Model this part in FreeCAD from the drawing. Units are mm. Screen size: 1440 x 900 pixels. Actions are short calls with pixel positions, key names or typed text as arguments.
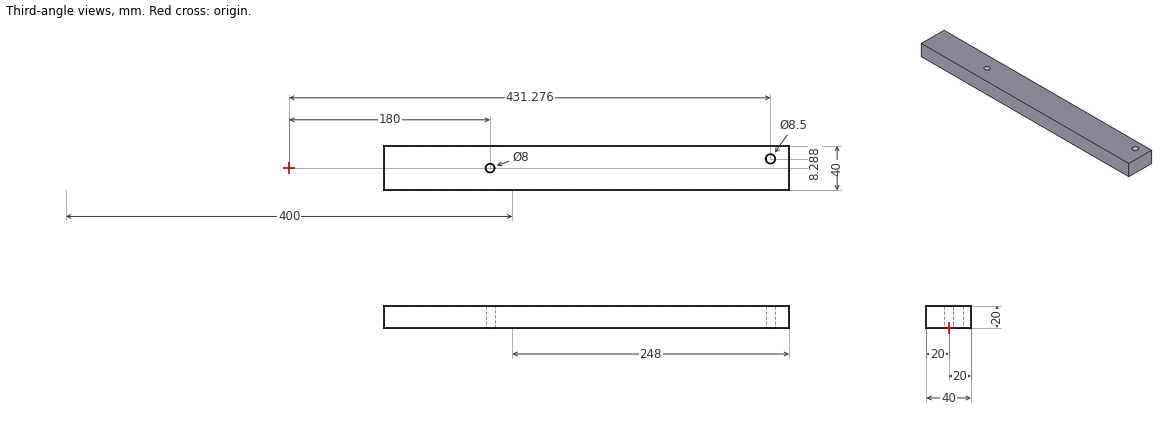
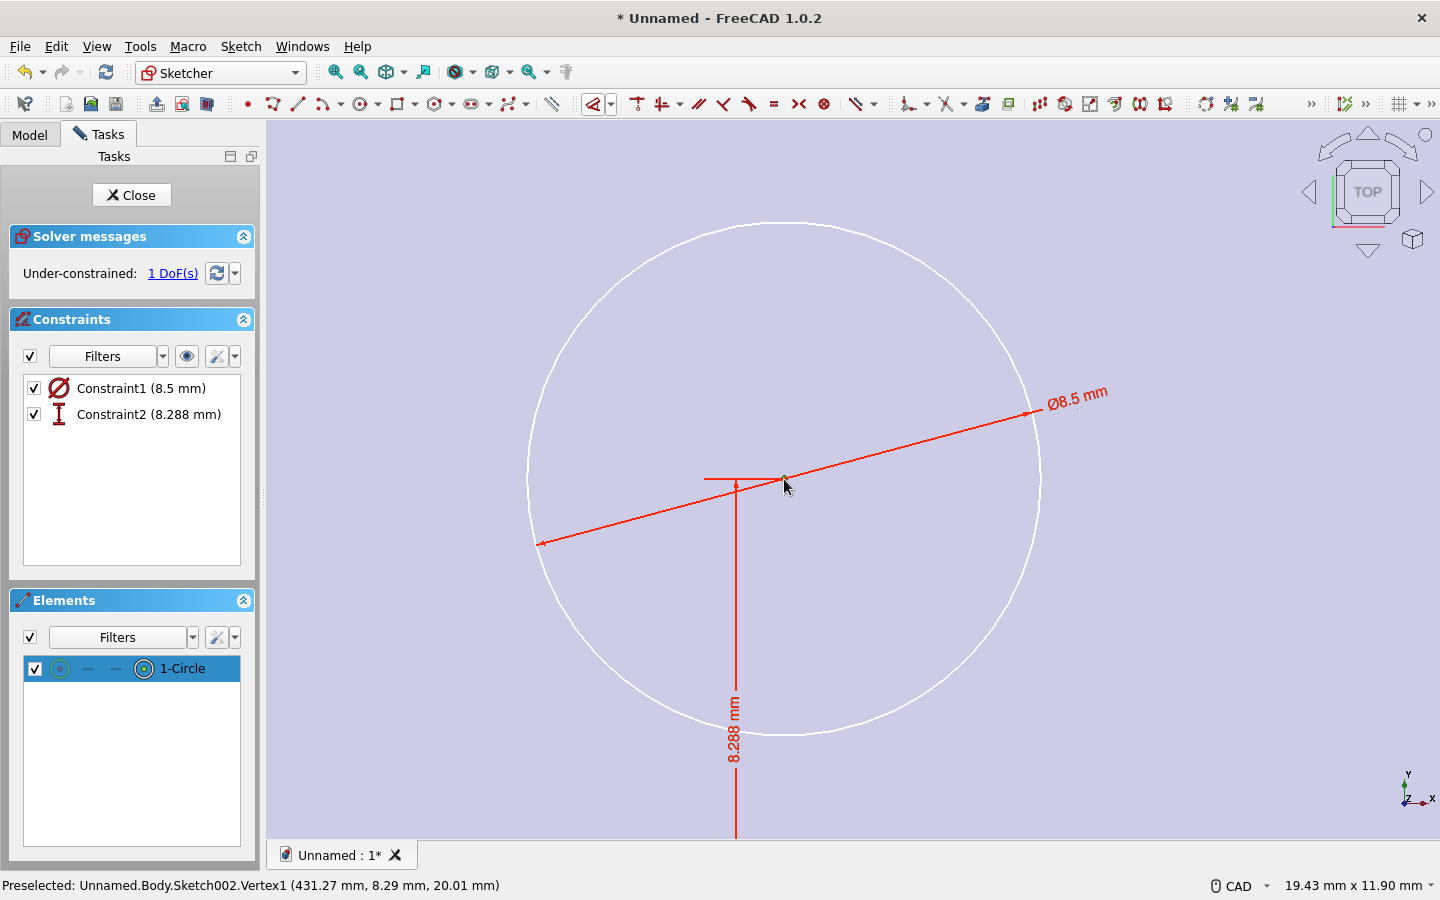
click(610, 104)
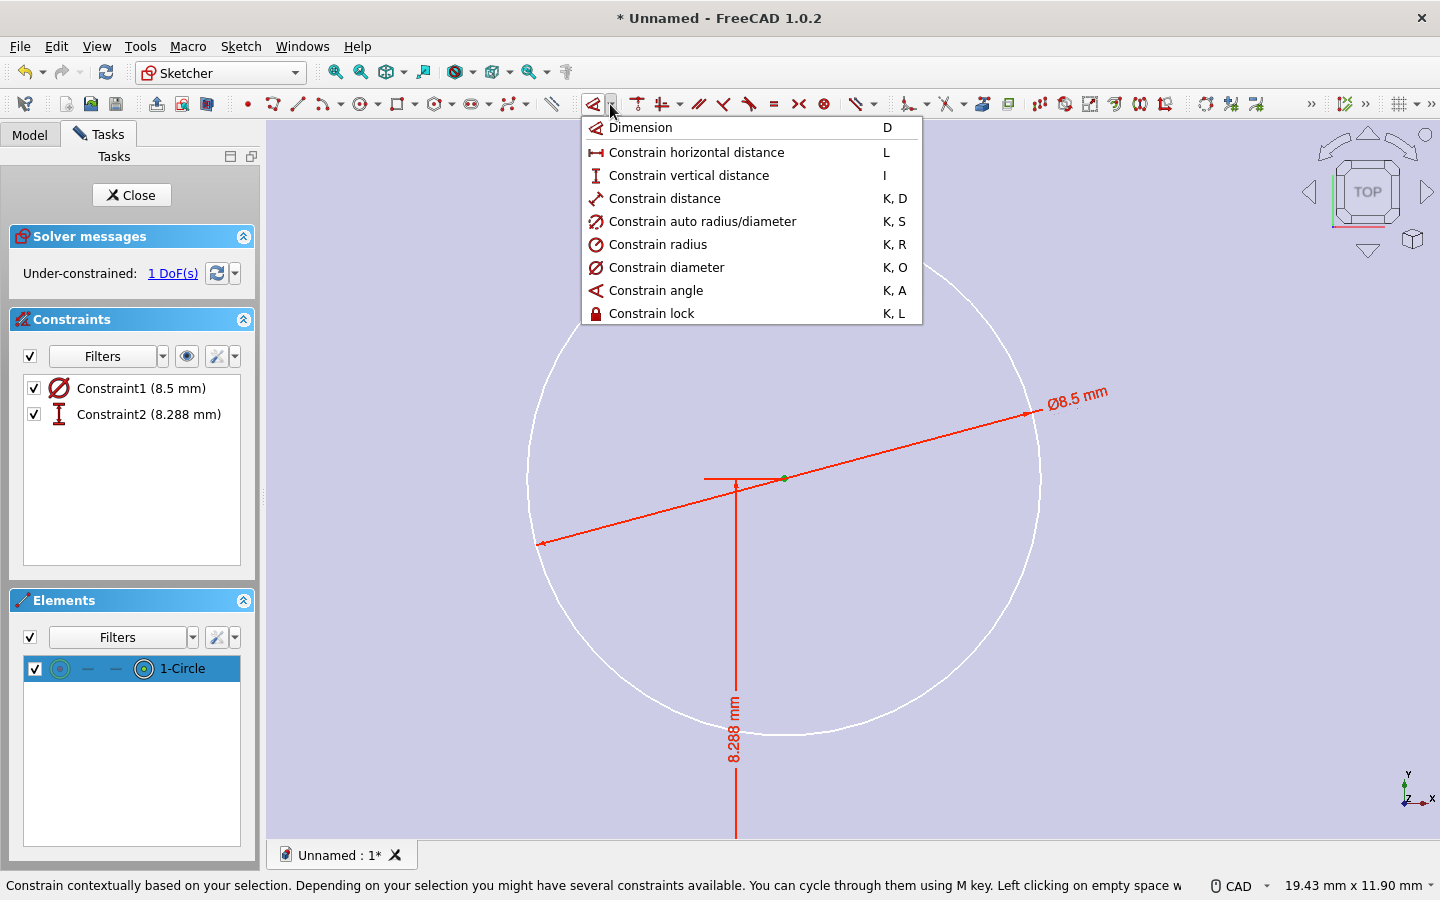
click(752, 152)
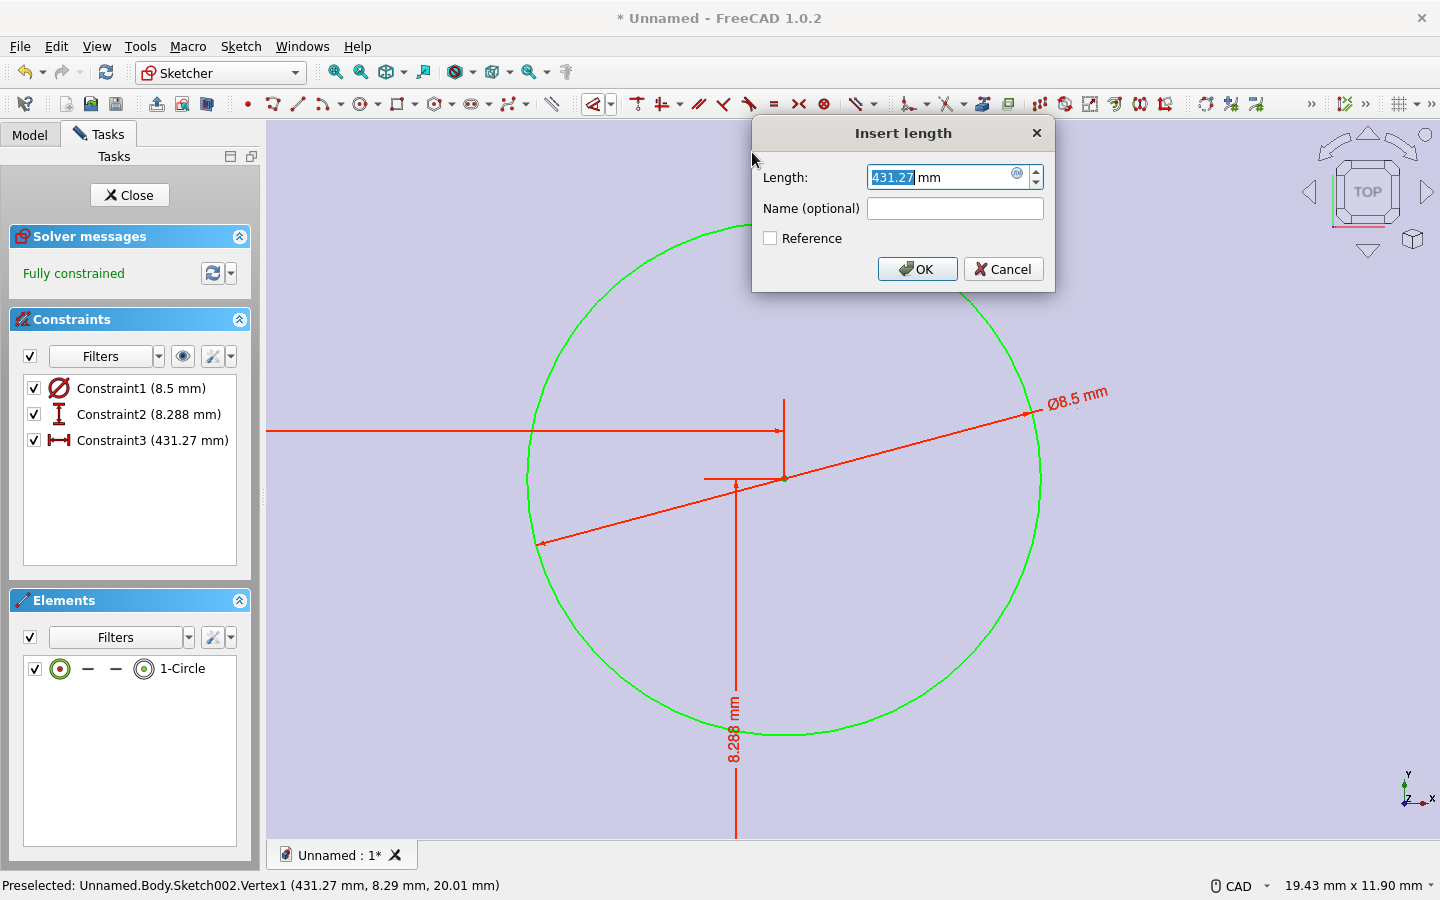
text(431.276)
key(Return)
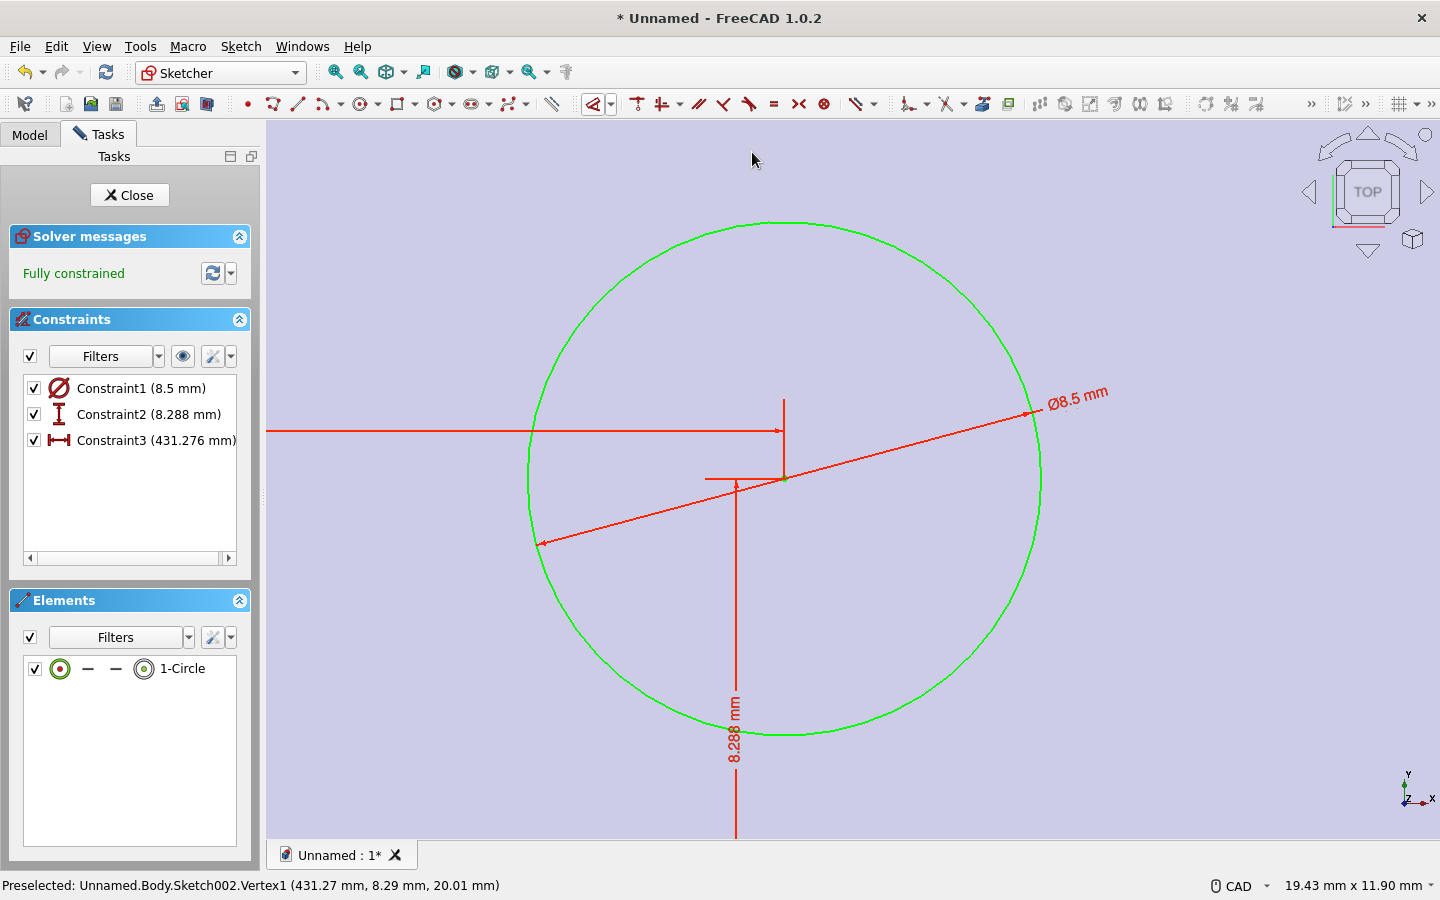
click(130, 195)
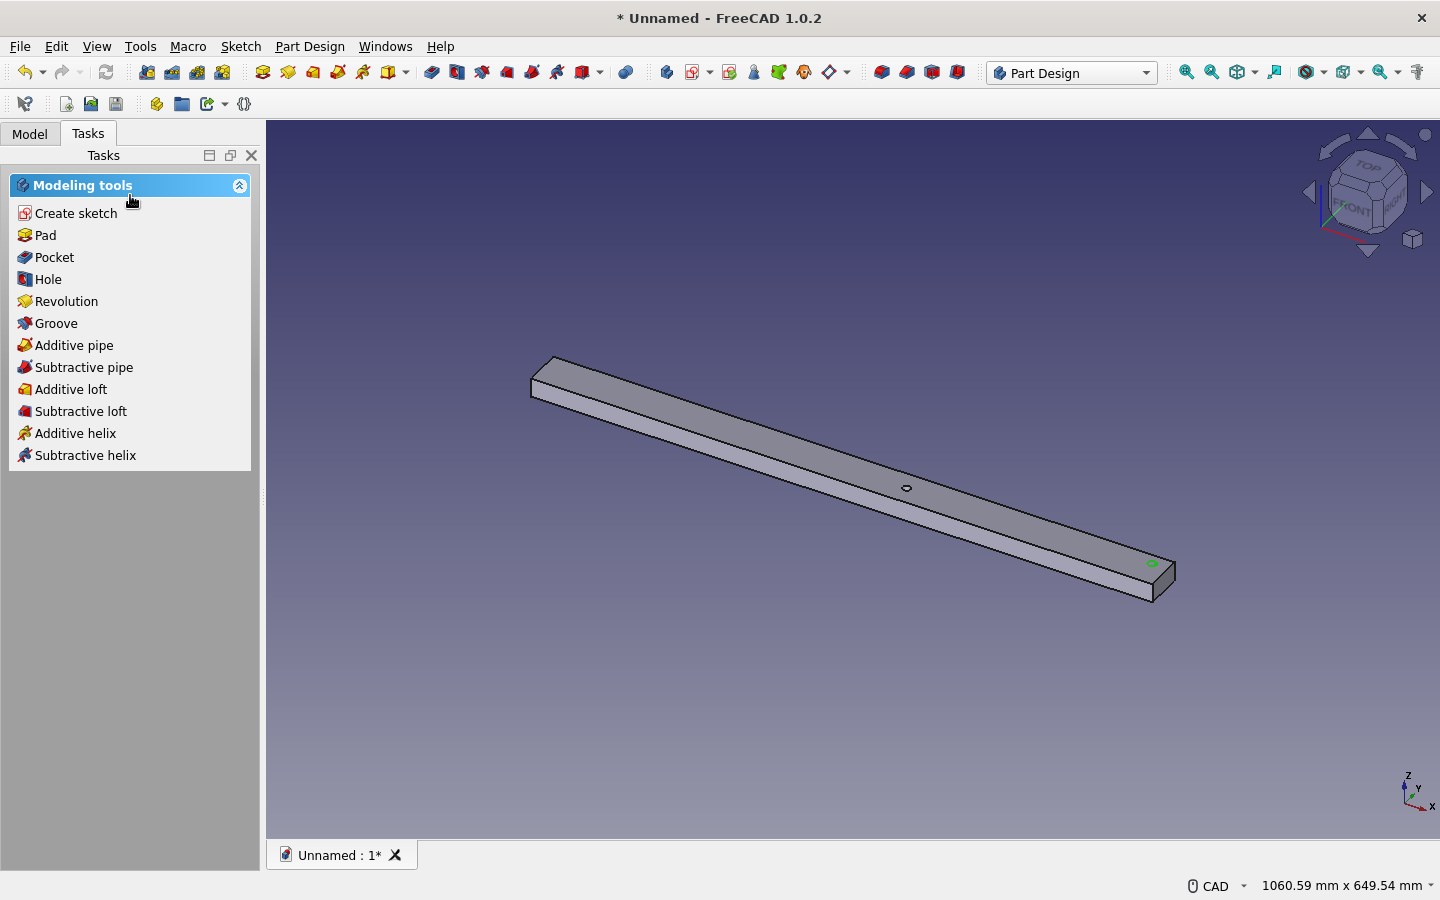
click(432, 72)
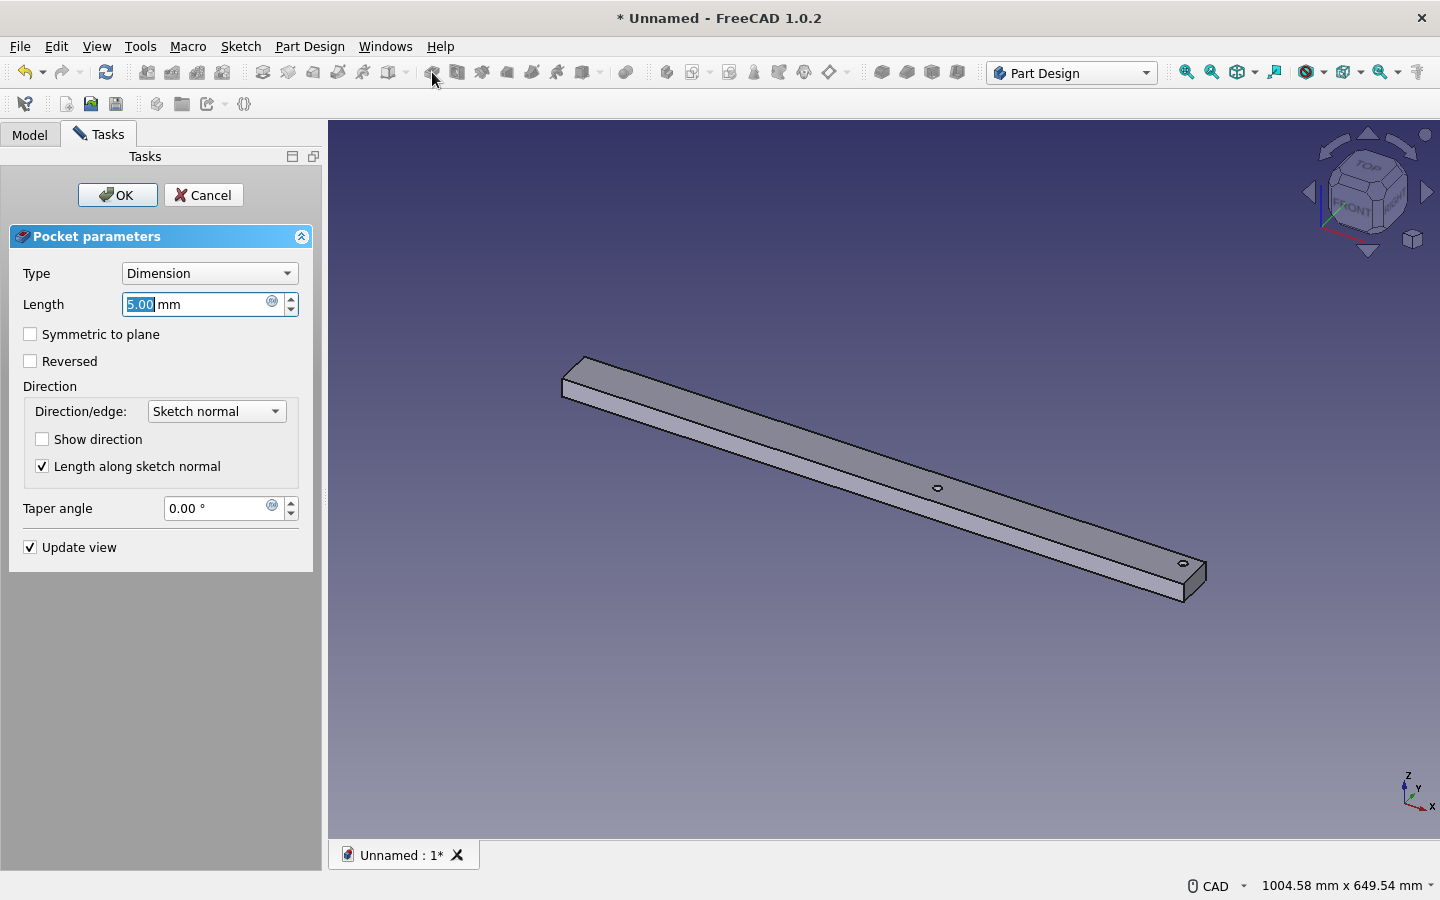
click(210, 274)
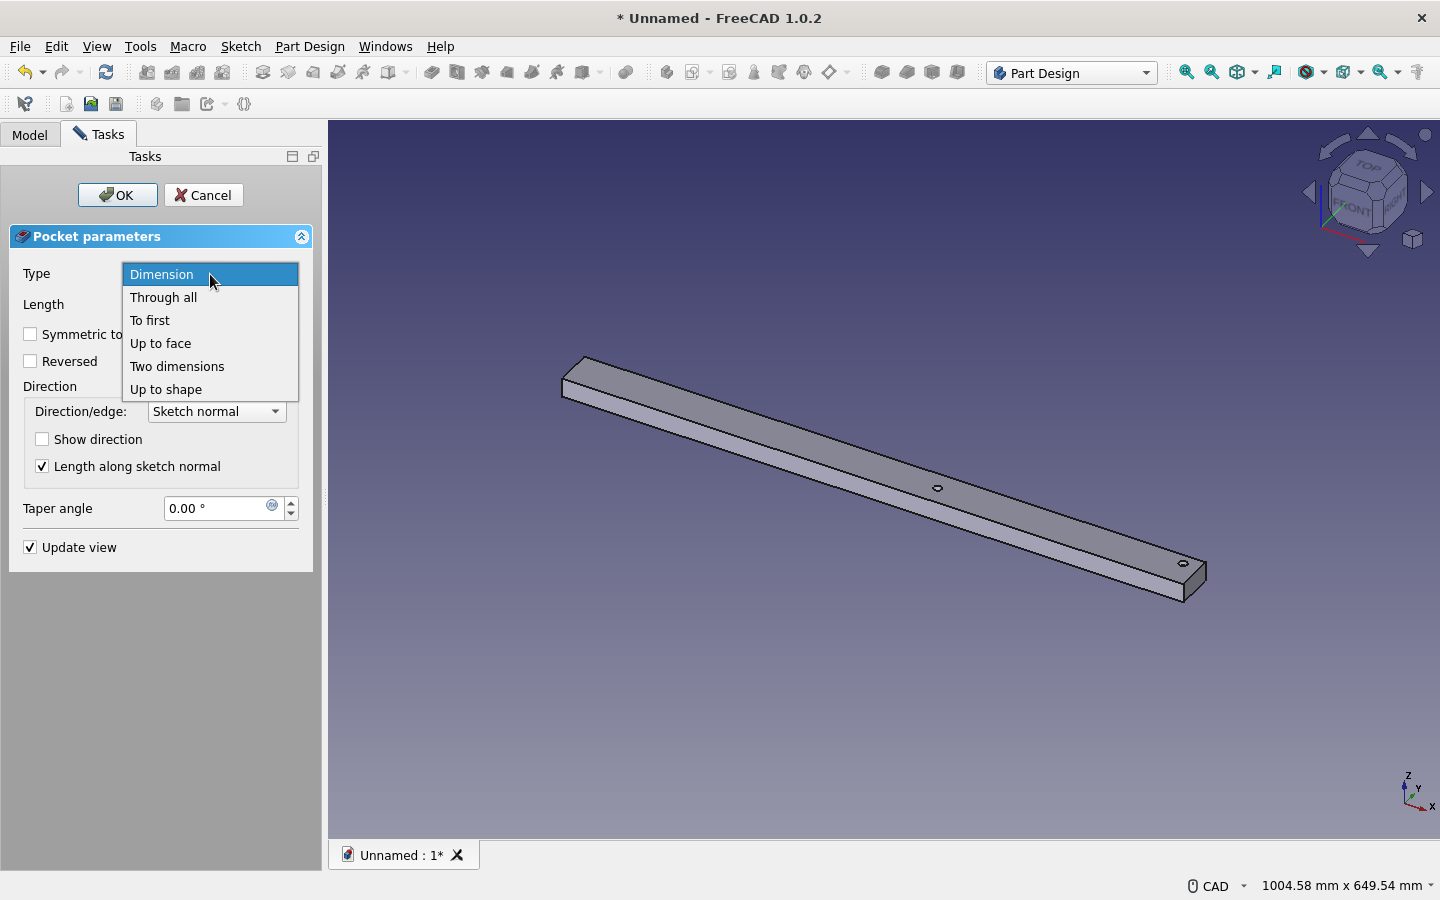
click(208, 298)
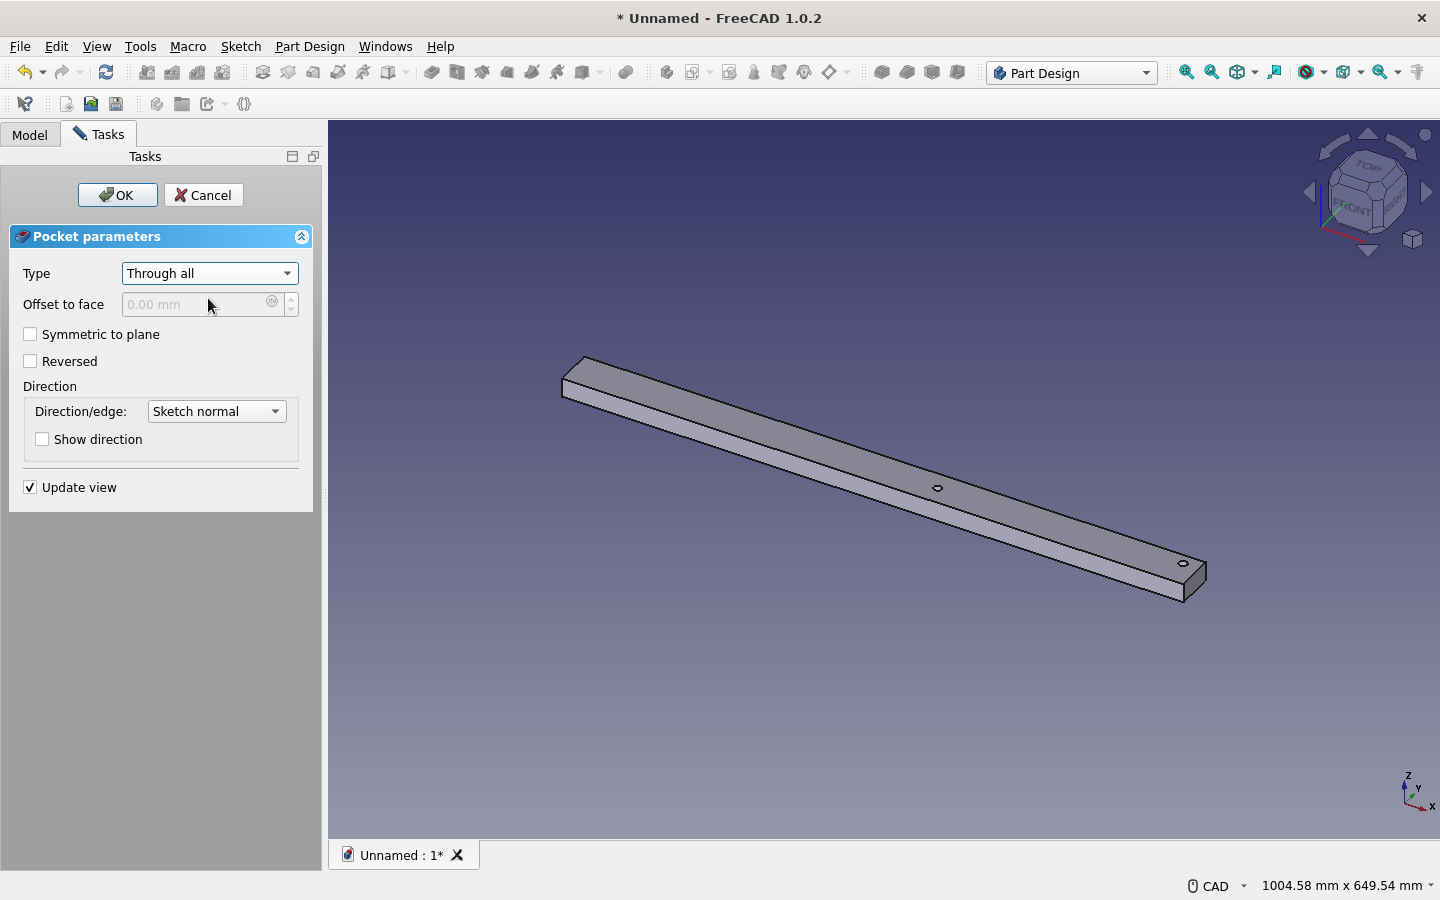
click(118, 195)